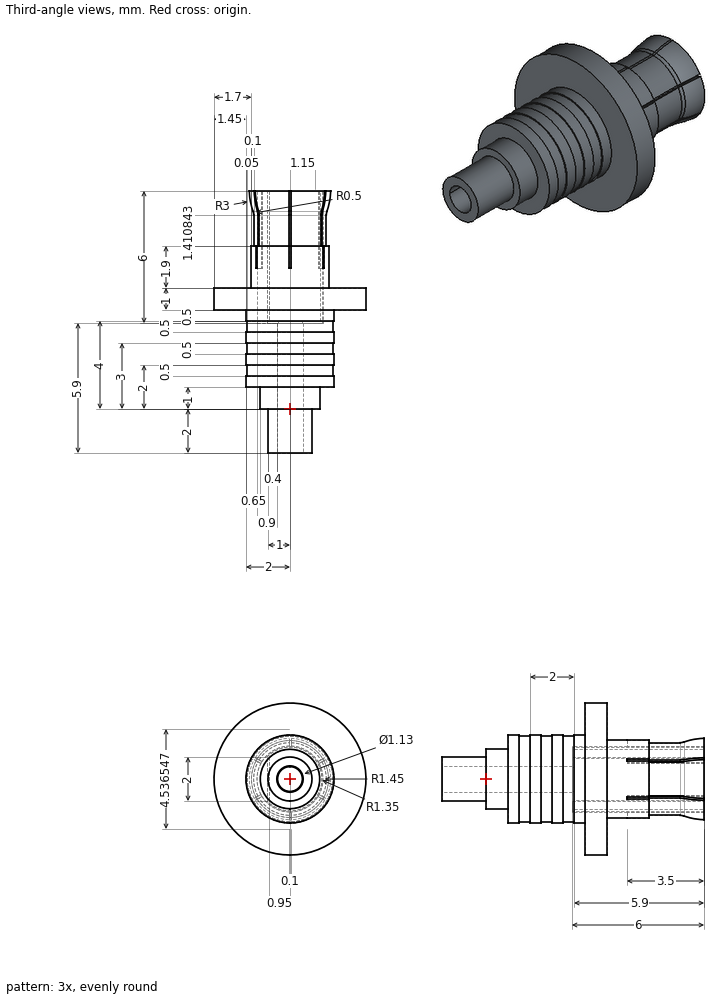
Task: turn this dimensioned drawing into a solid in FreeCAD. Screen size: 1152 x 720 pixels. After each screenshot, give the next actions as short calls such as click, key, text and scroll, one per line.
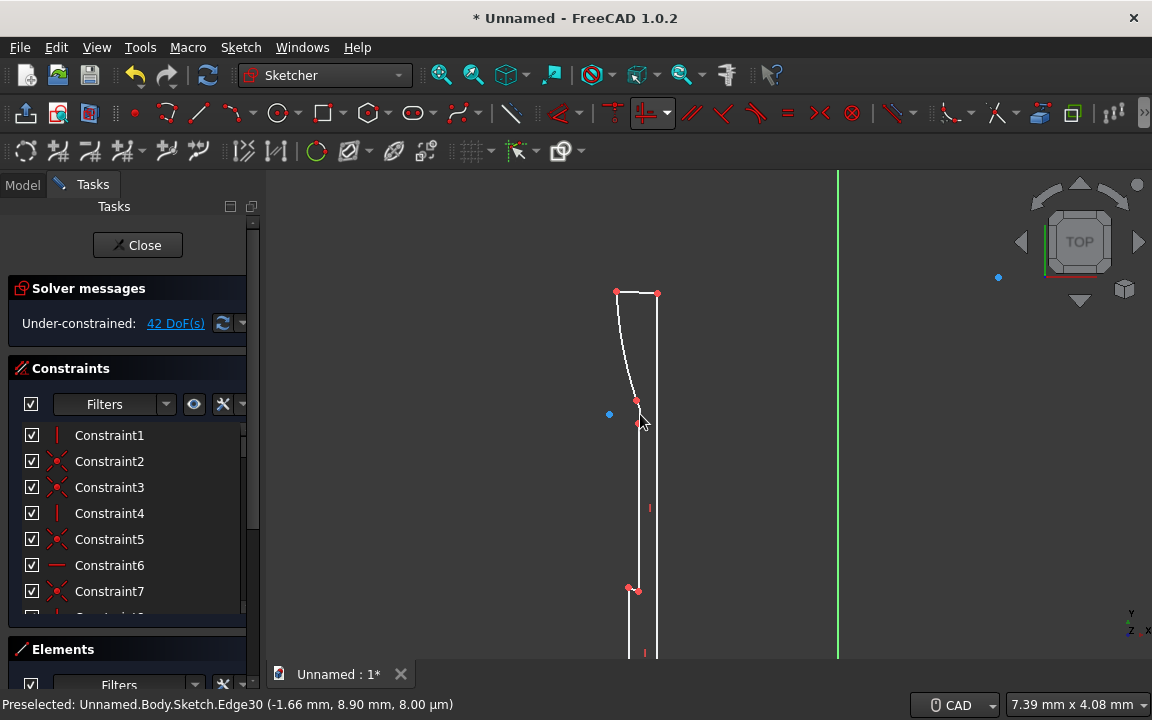
scroll(643, 266, down, 8)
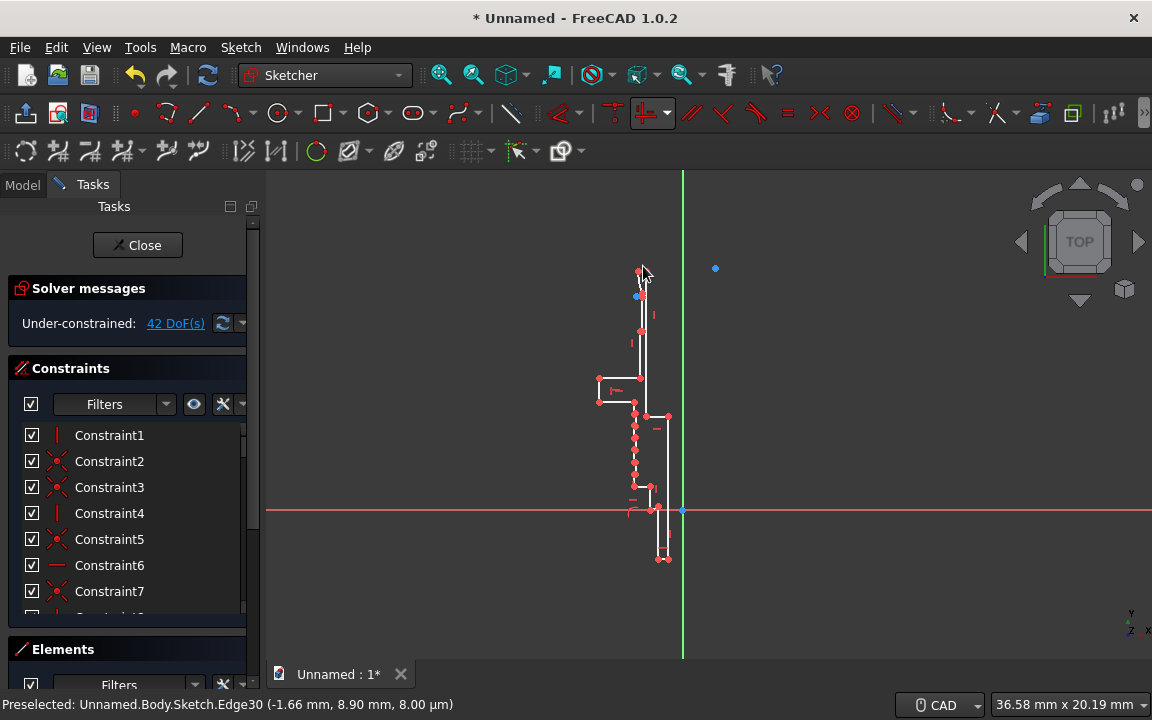
scroll(642, 308, up, 7)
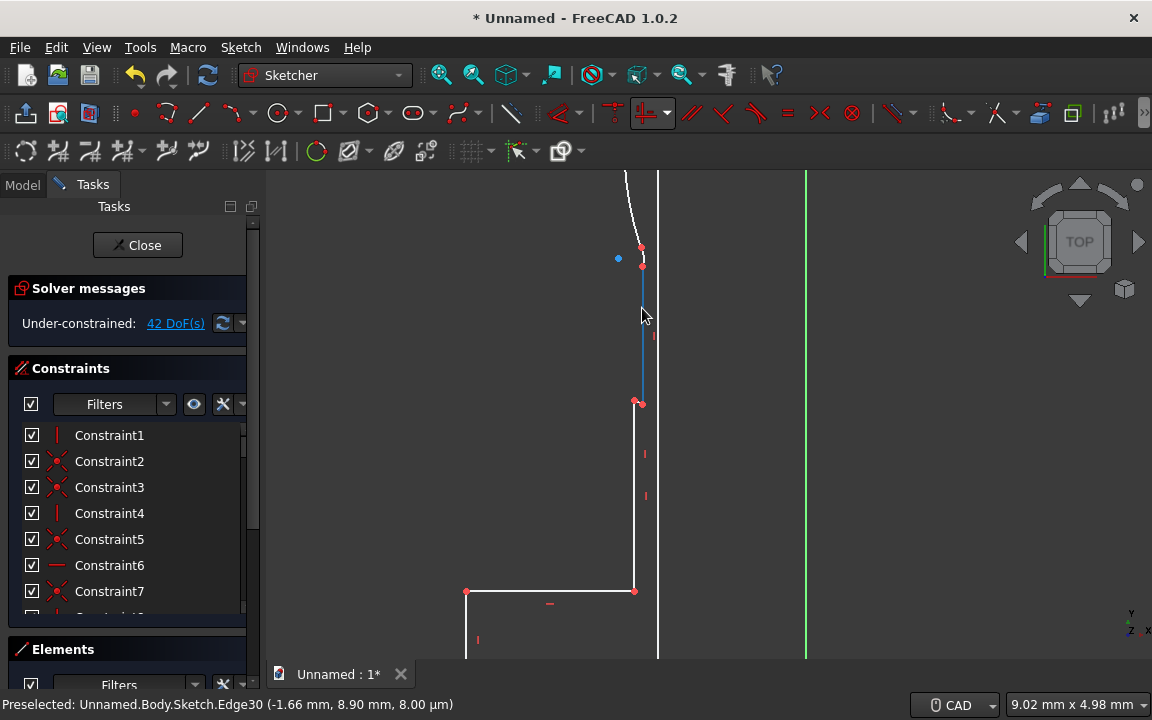
click(643, 308)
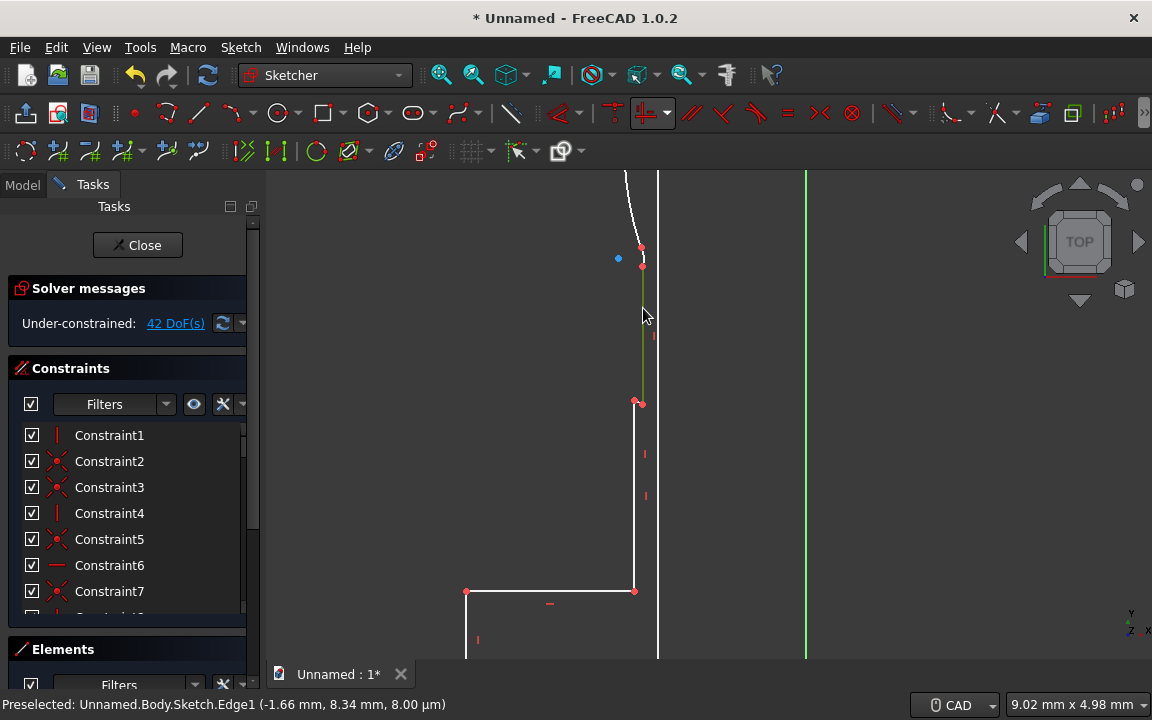
scroll(644, 257, up, 2)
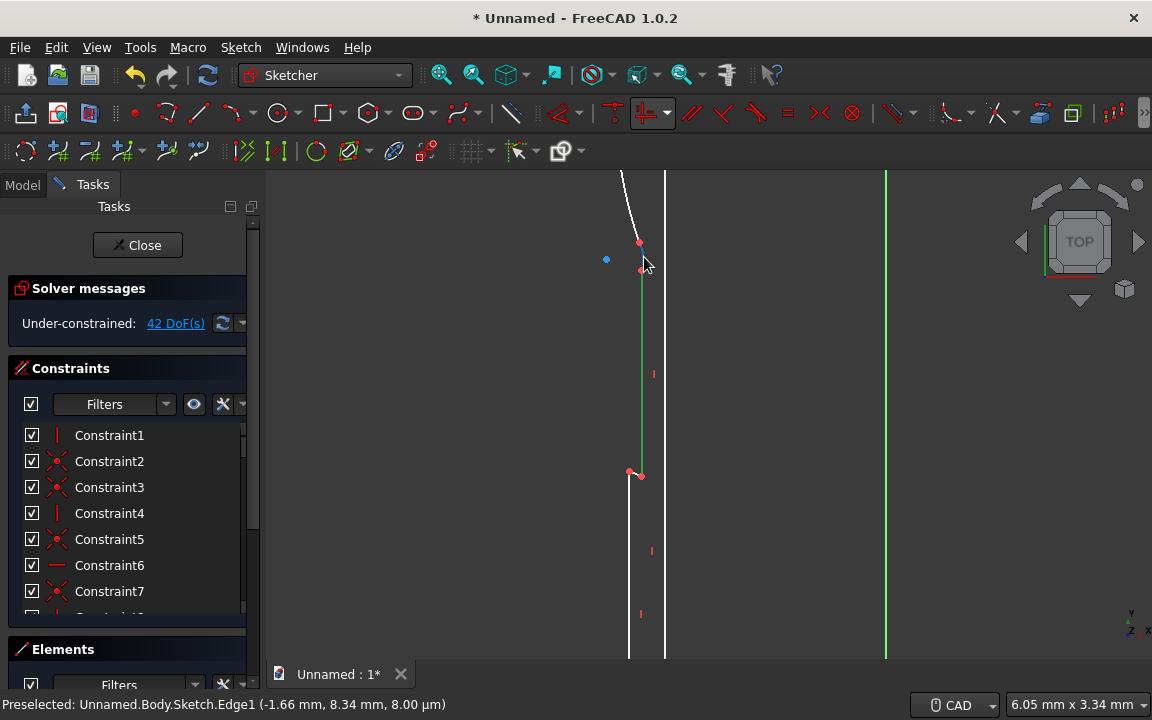
click(643, 257)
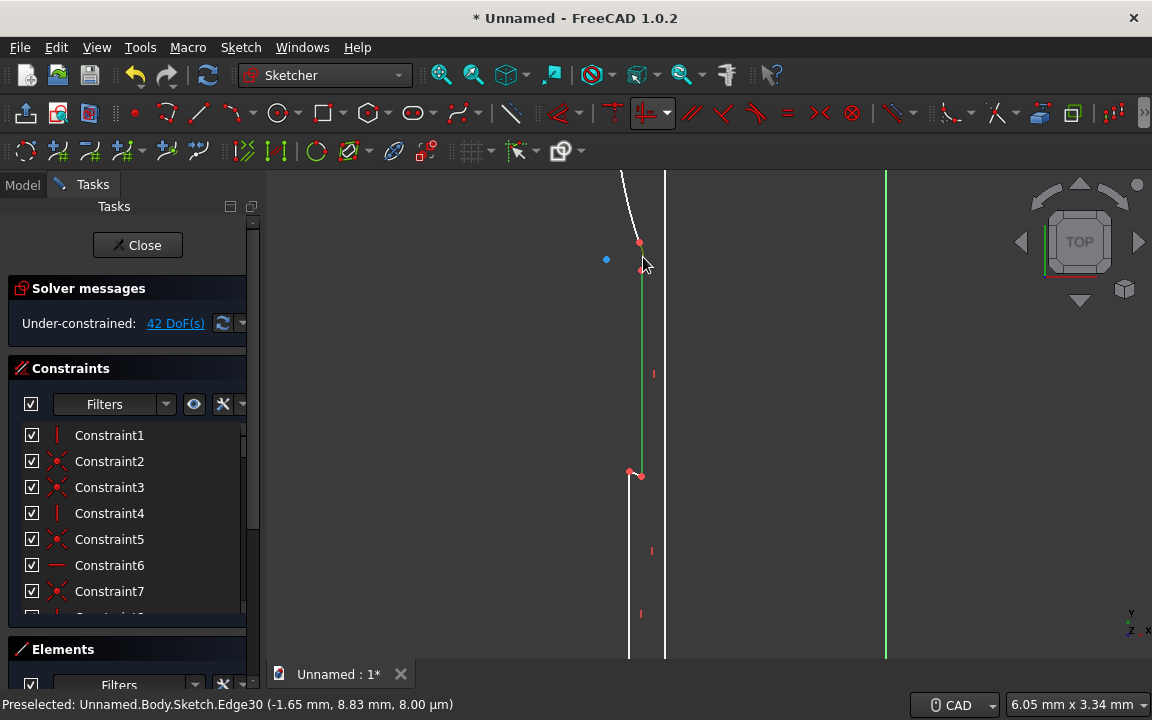
click(756, 114)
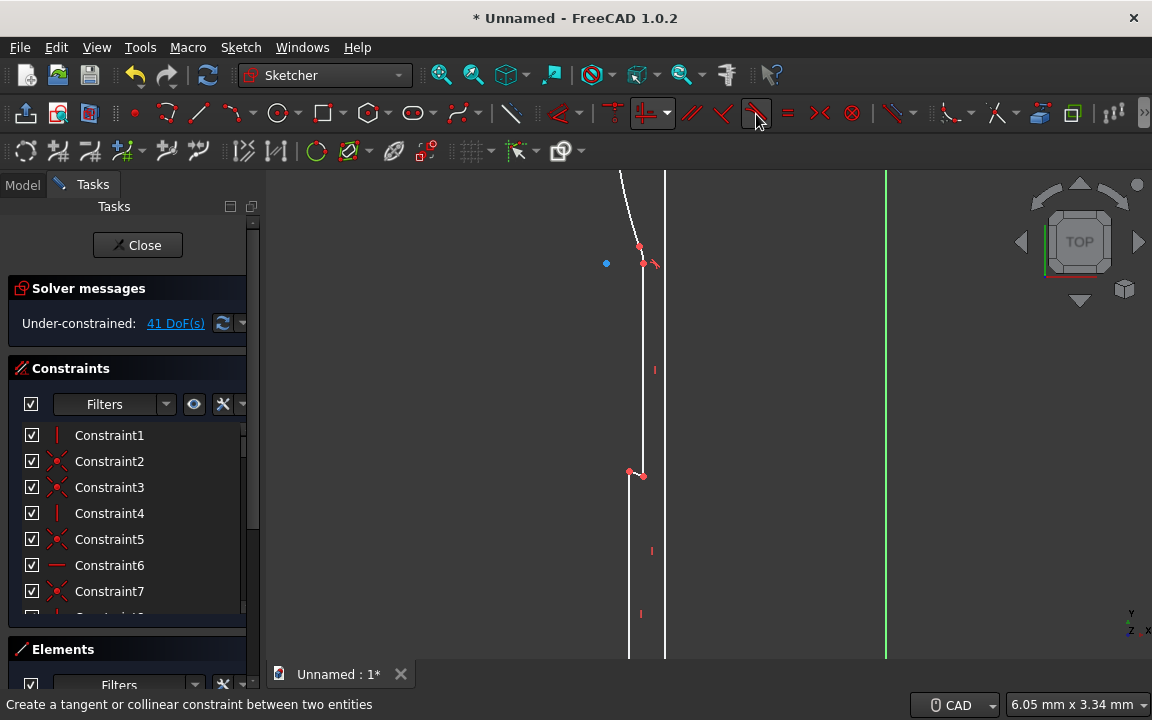
click(627, 206)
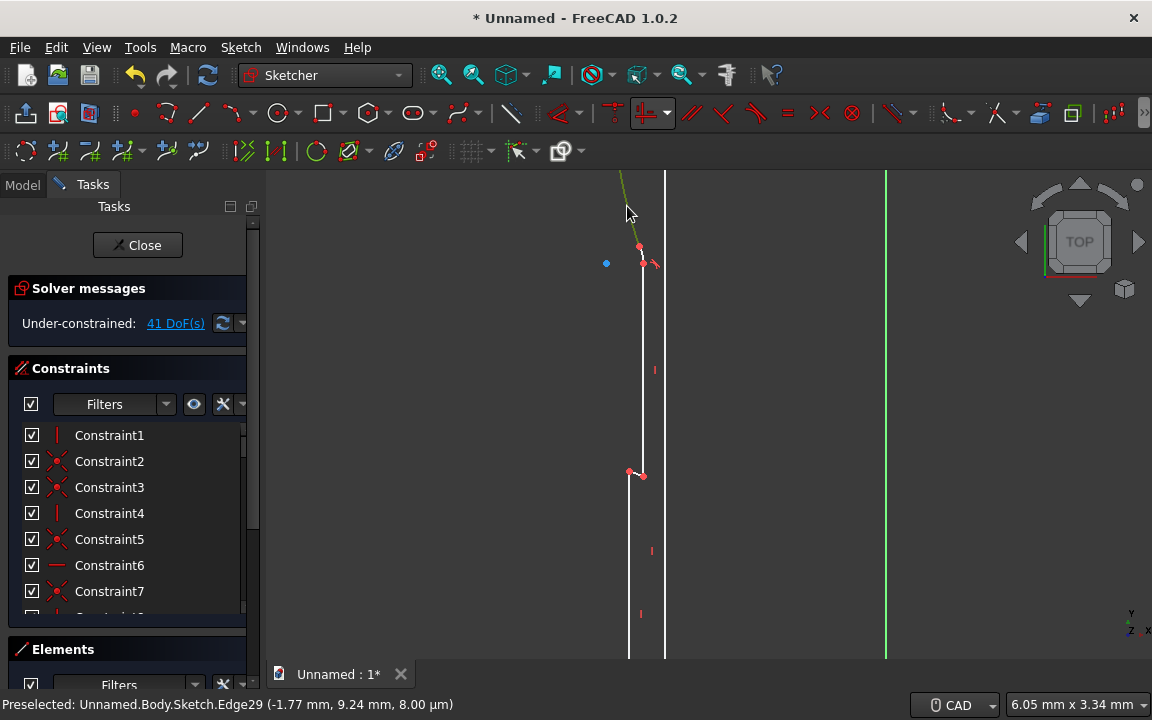
scroll(642, 255, up, 3)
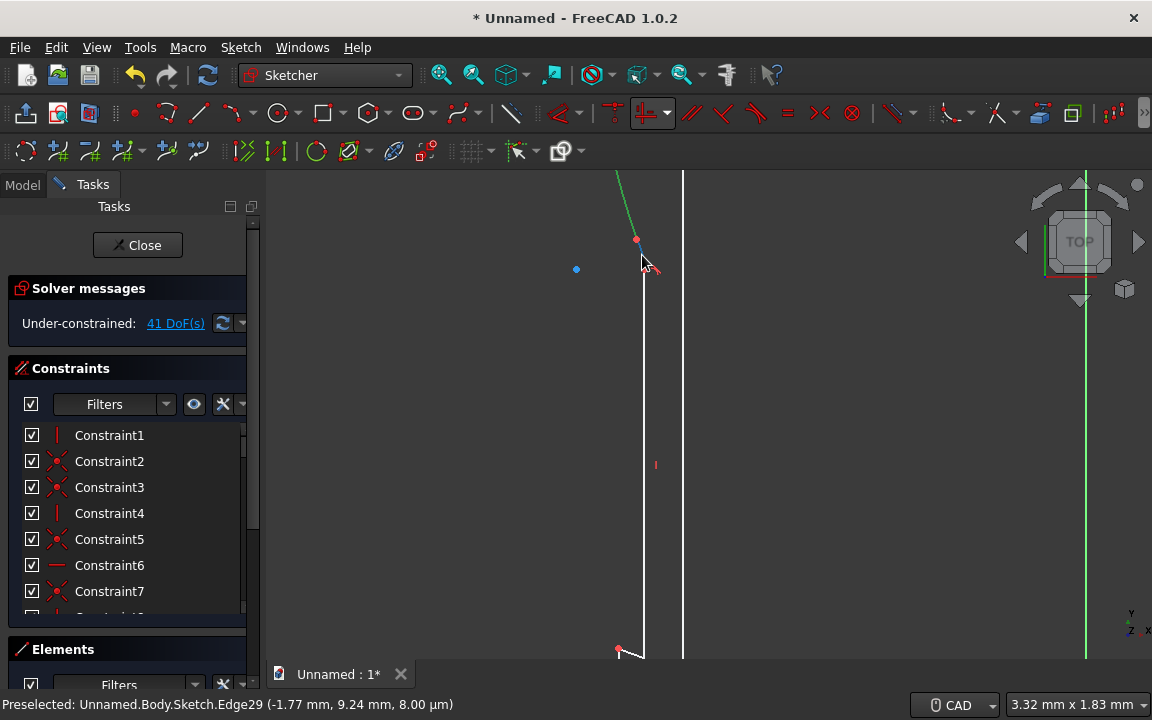
click(642, 254)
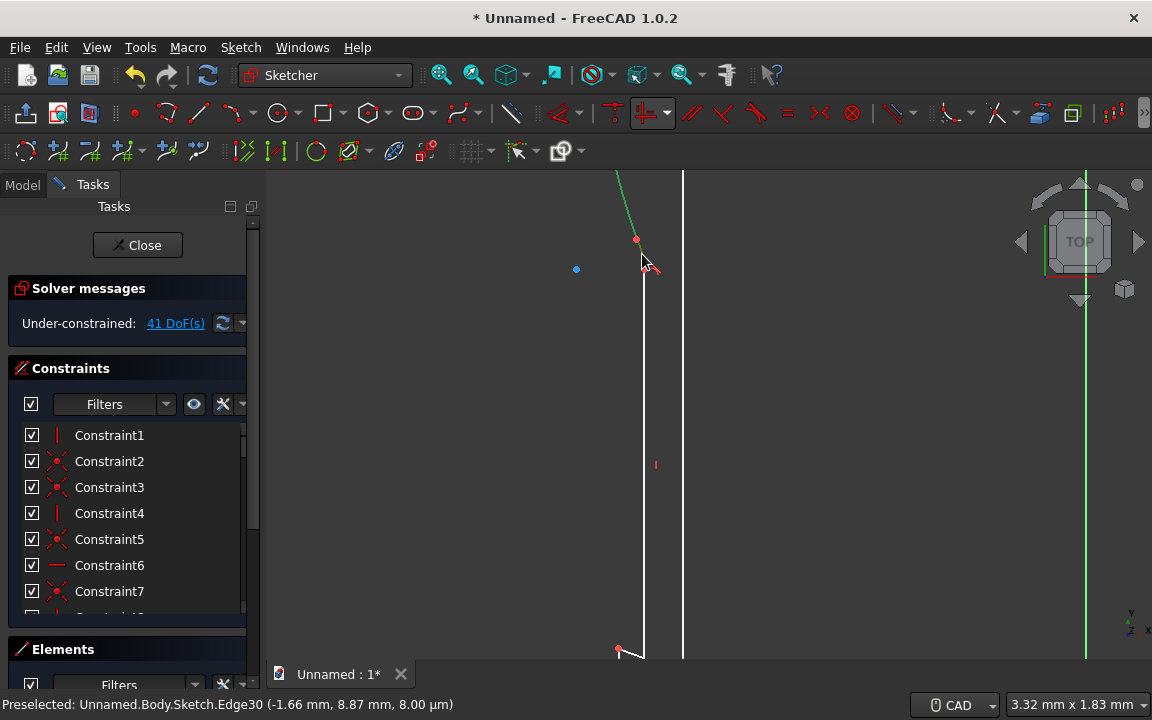
click(756, 114)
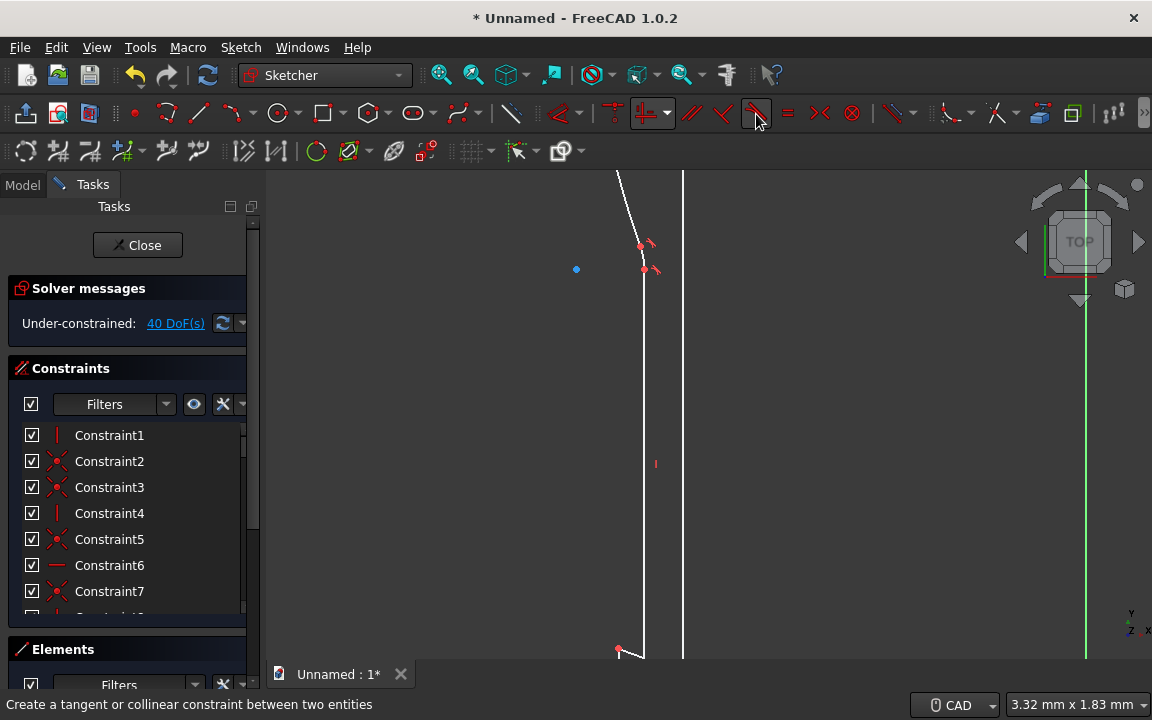
scroll(642, 299, down, 12)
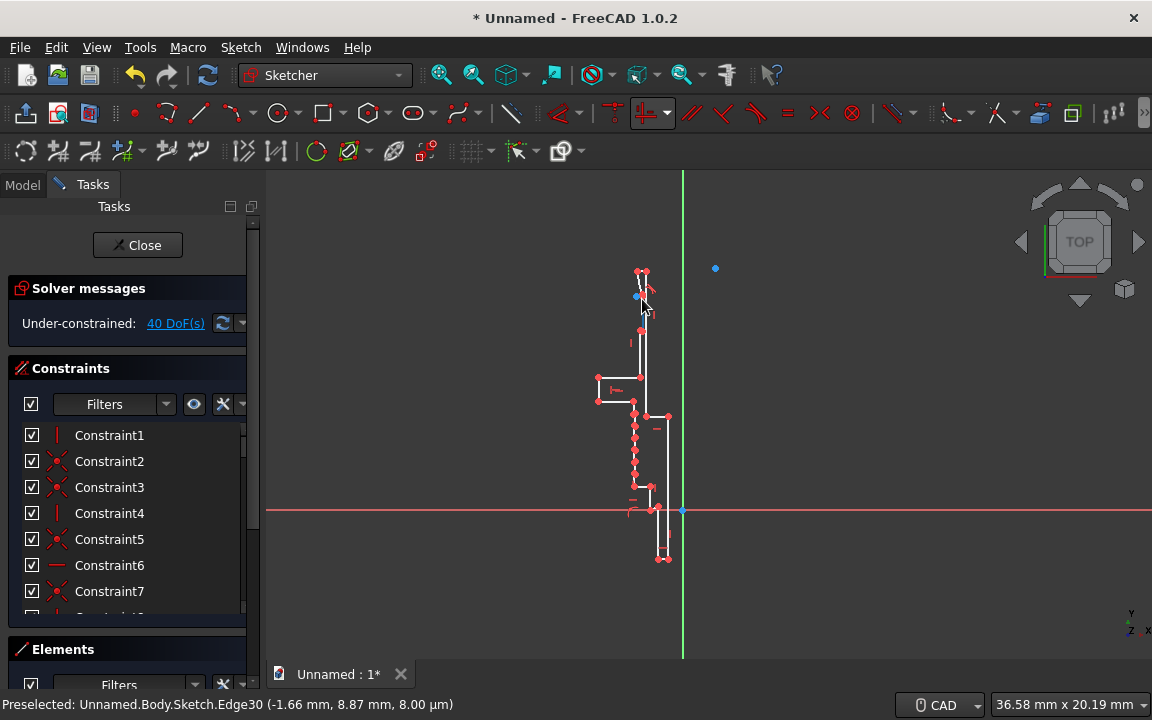
scroll(642, 331, up, 14)